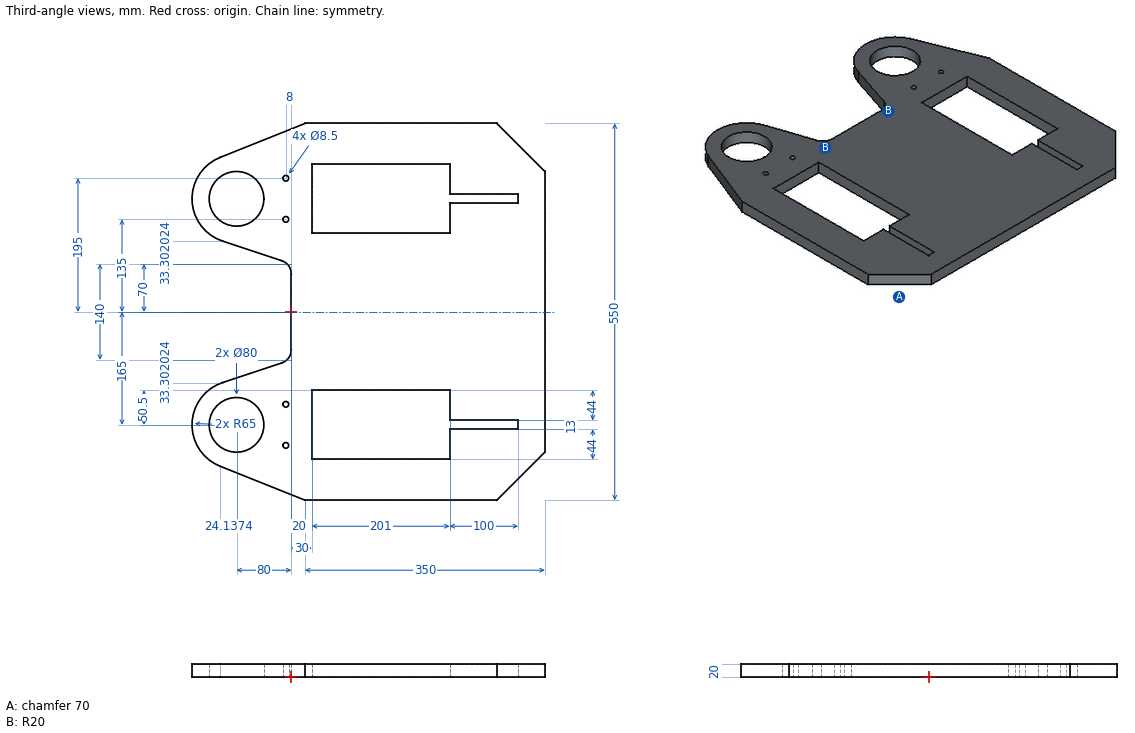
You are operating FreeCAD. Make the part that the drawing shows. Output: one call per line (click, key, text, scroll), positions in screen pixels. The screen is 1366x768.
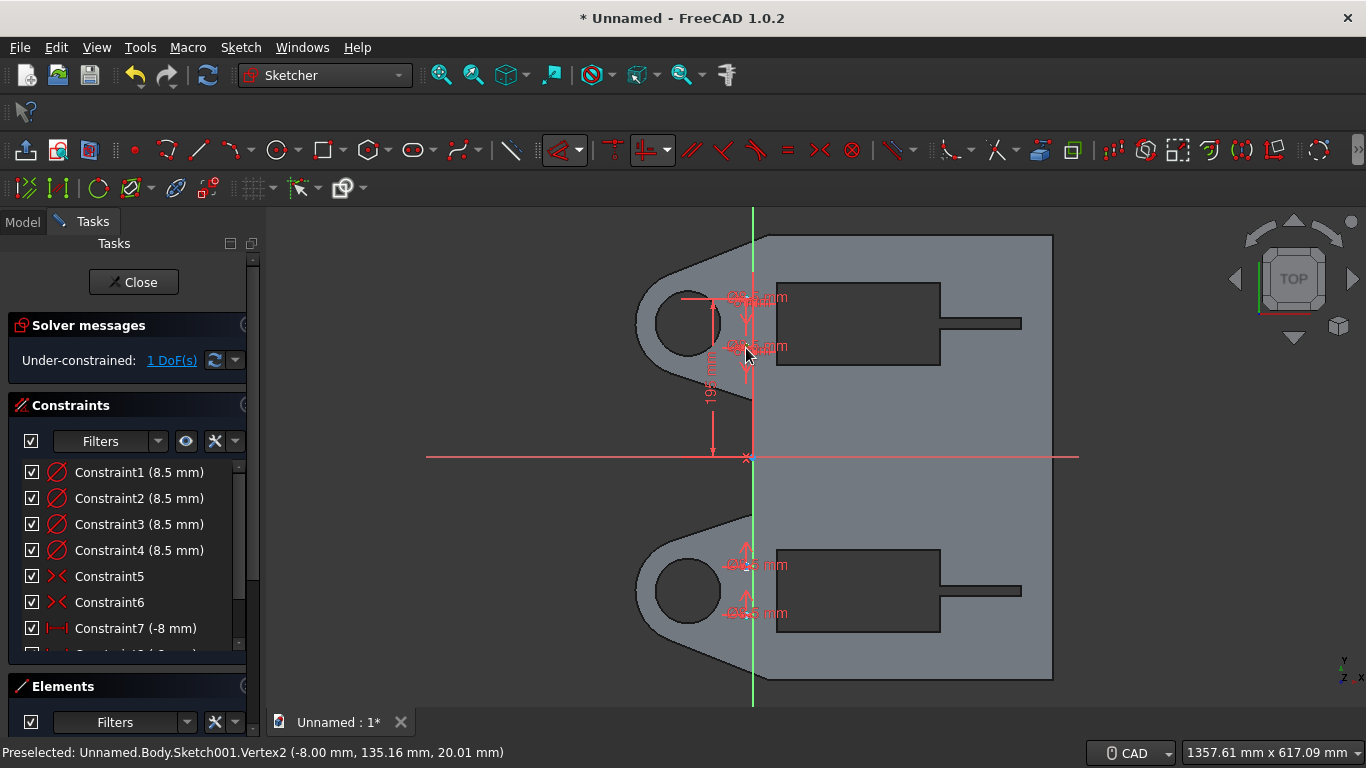
key(i)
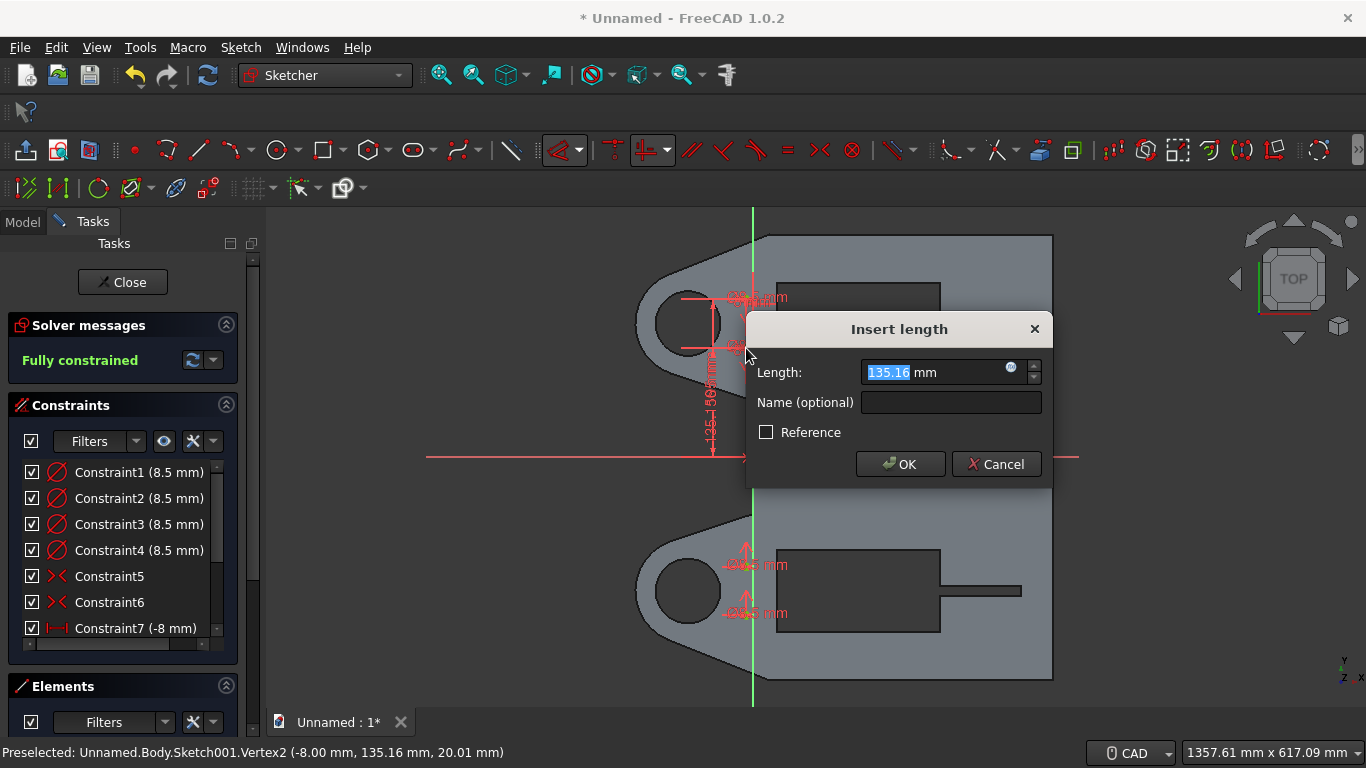
text(135)
key(Return)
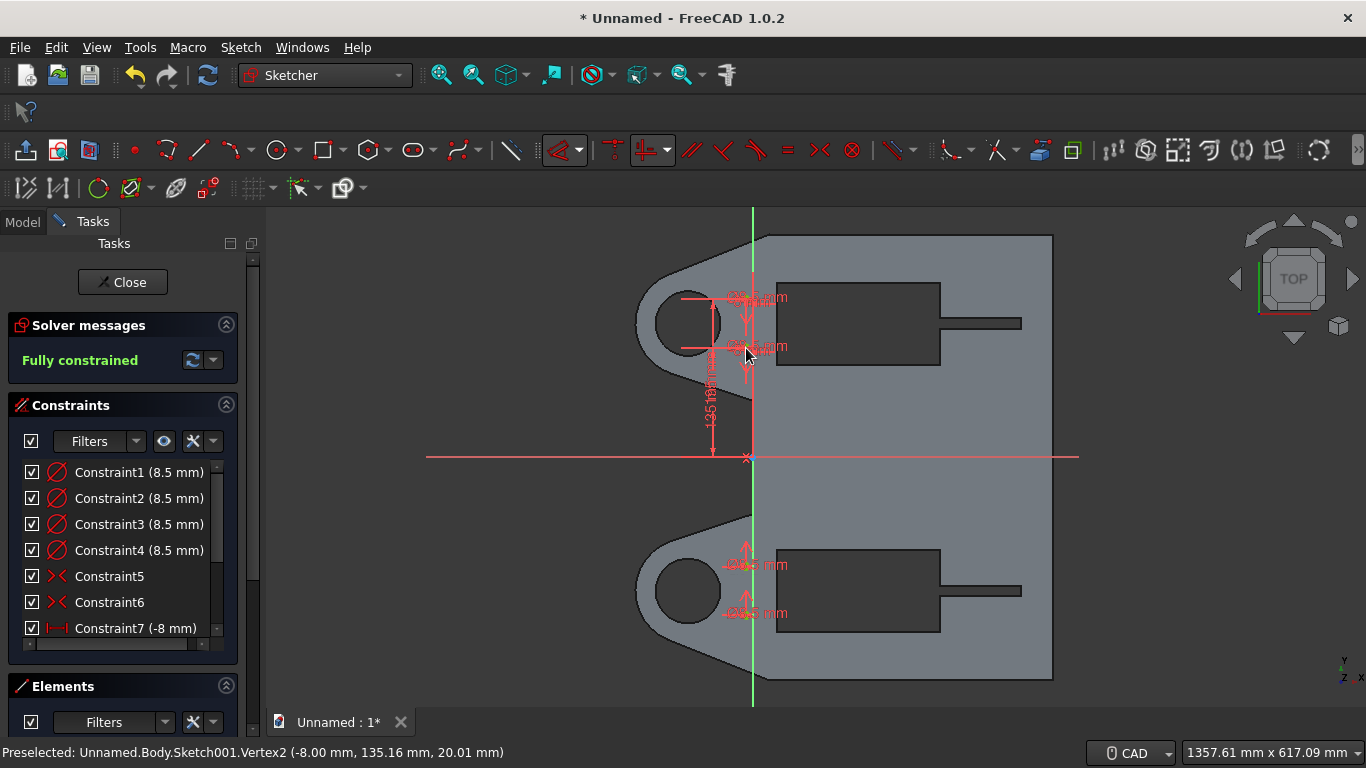
click(123, 282)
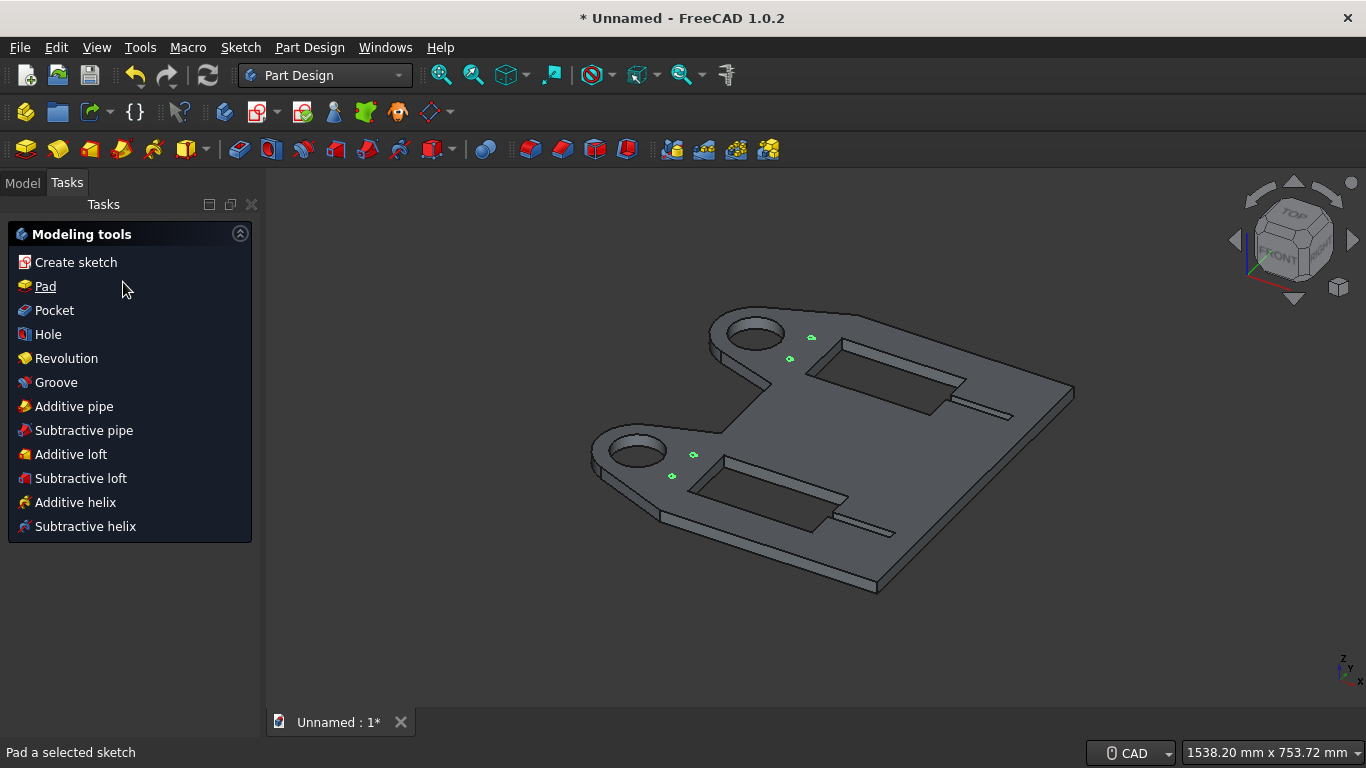
click(240, 150)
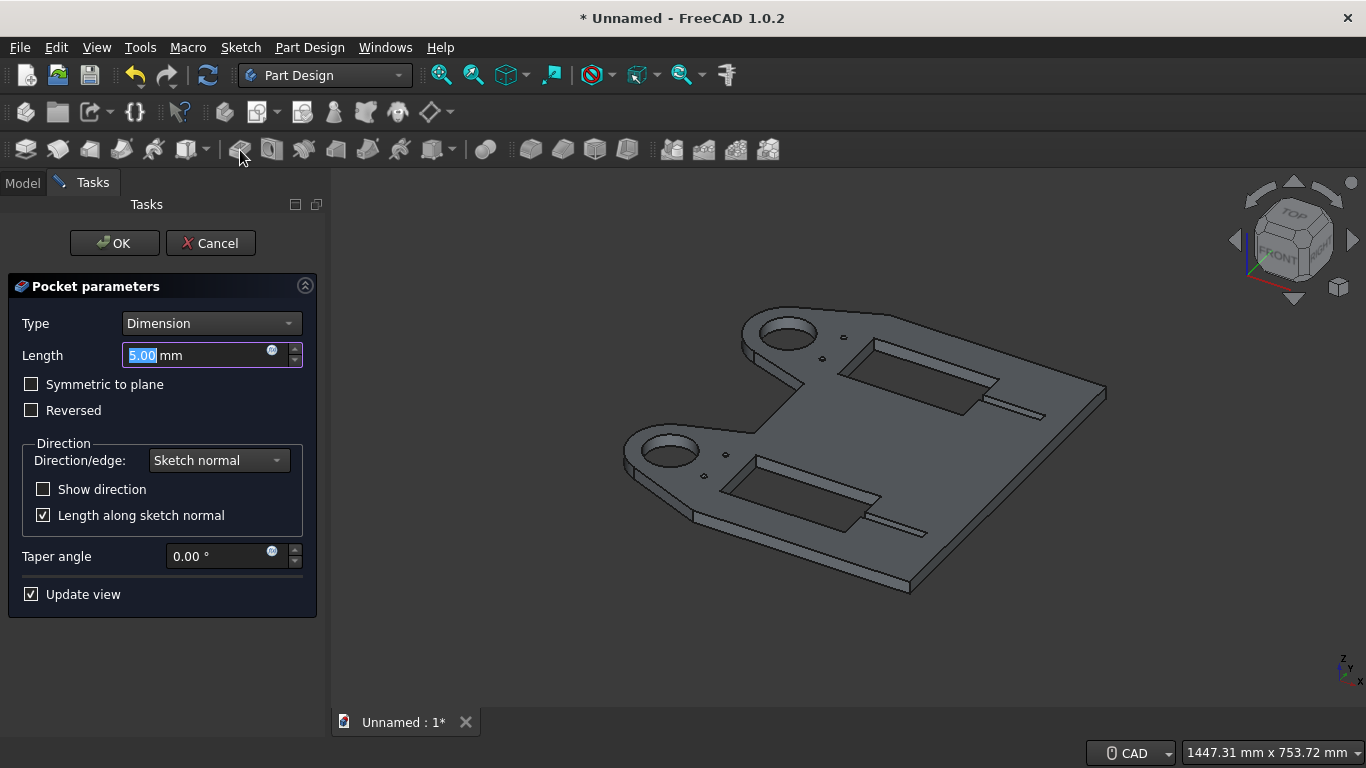
click(212, 324)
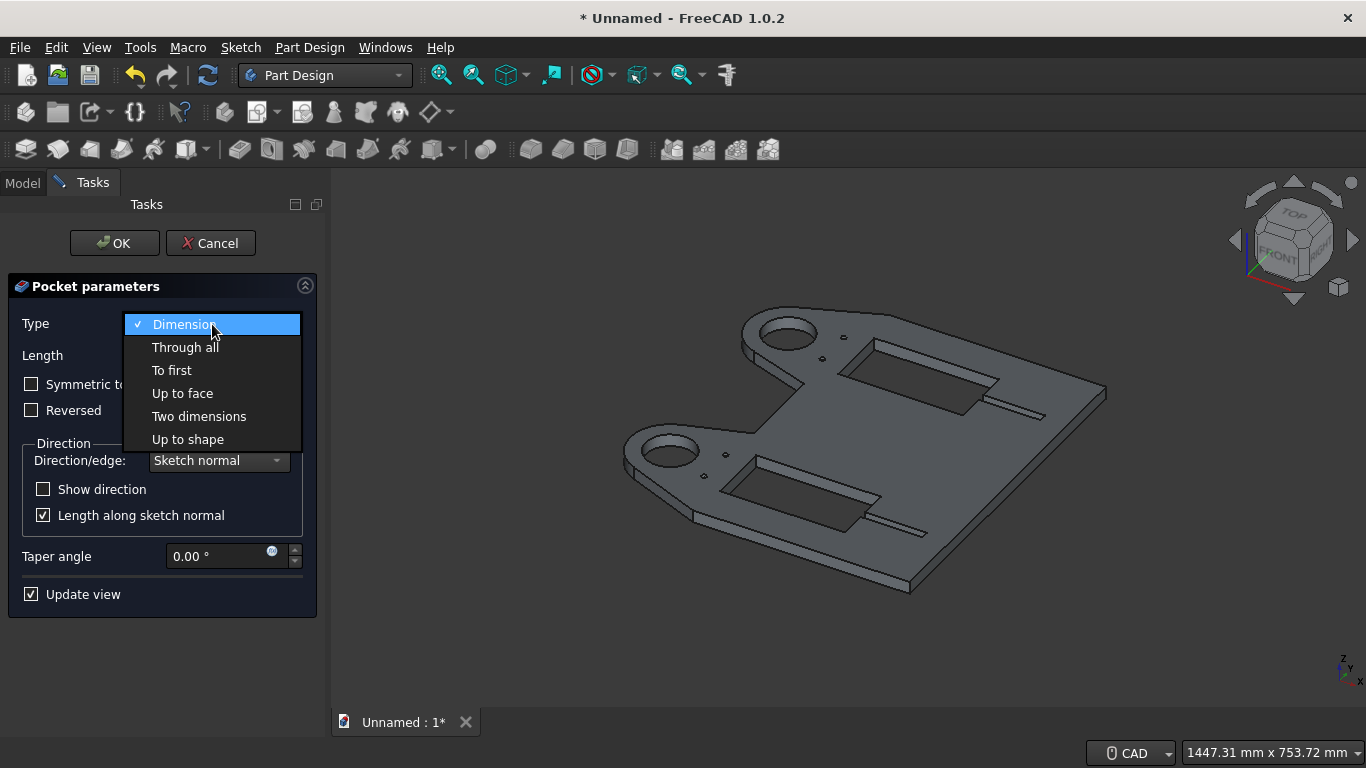
click(212, 348)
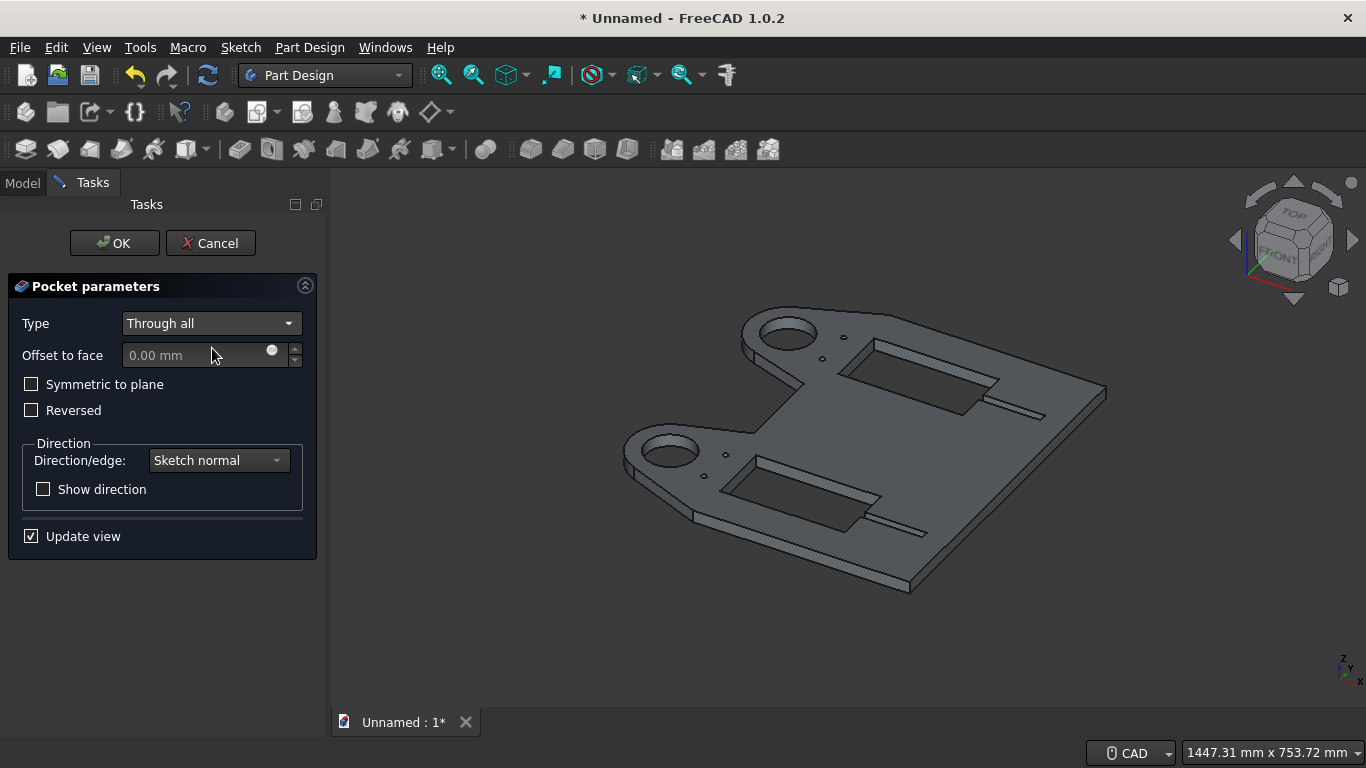
click(115, 243)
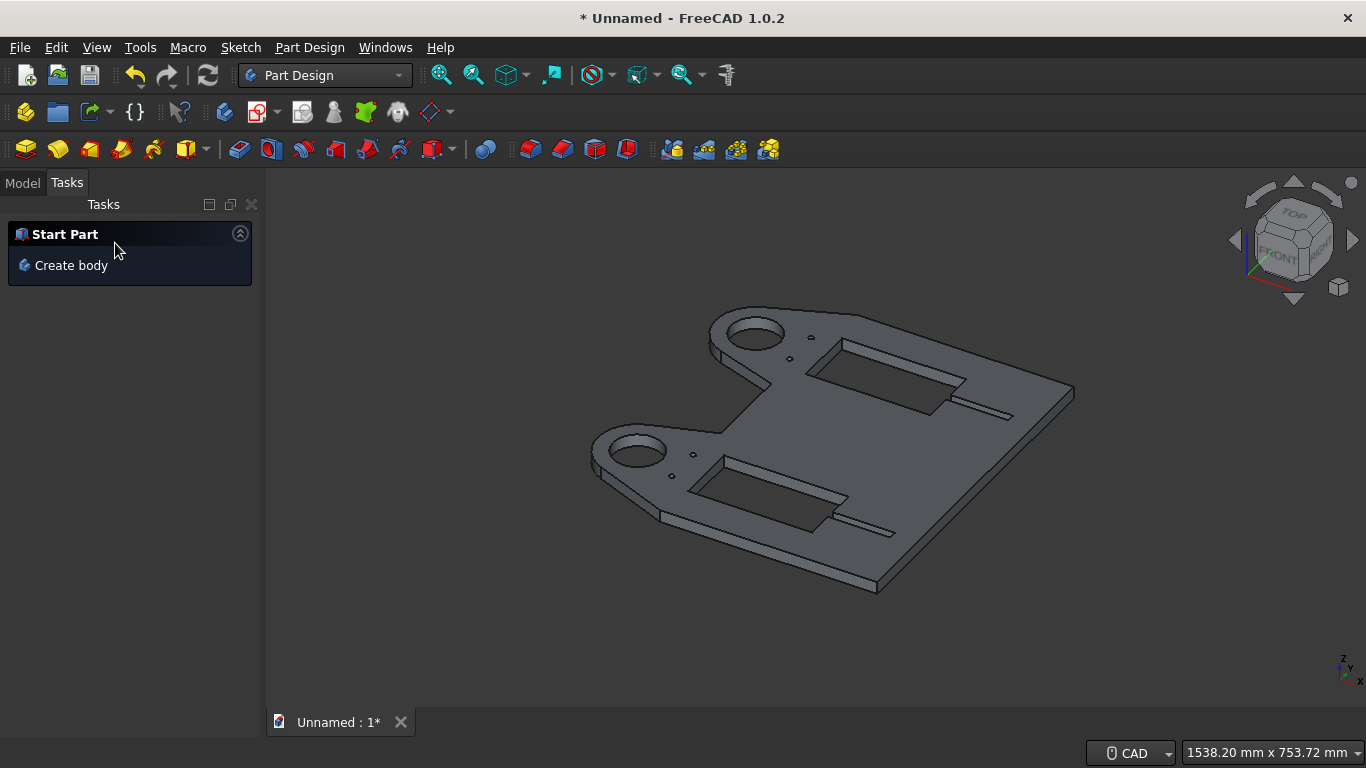
click(877, 588)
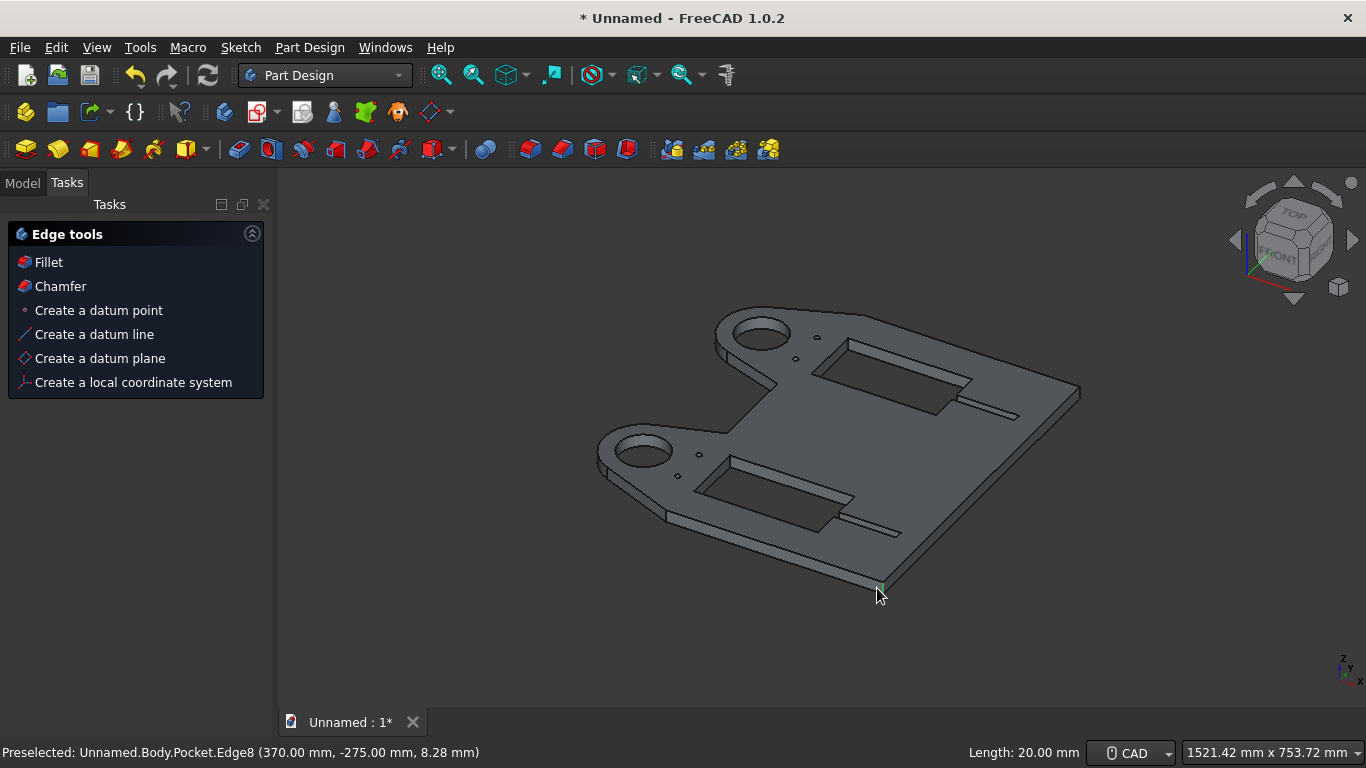
scroll(1080, 392, up, 6)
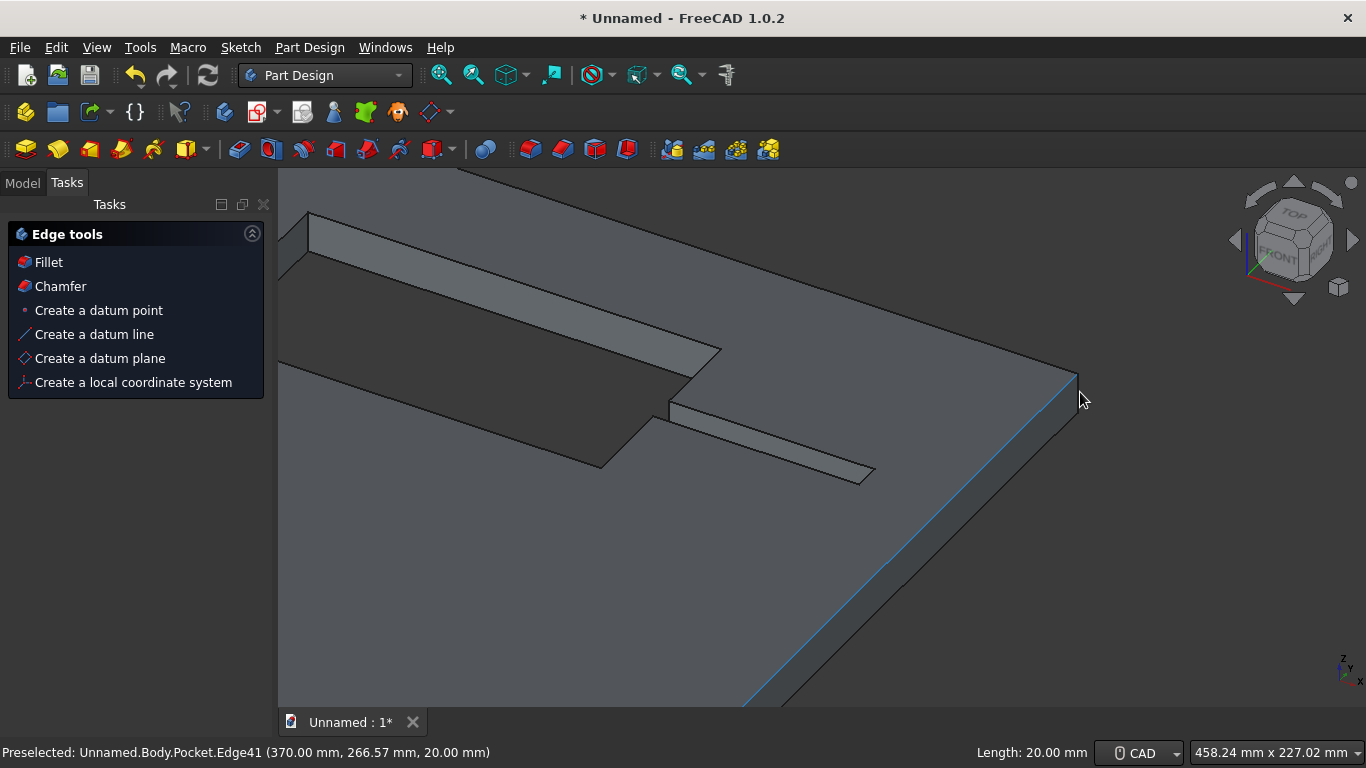
click(442, 76)